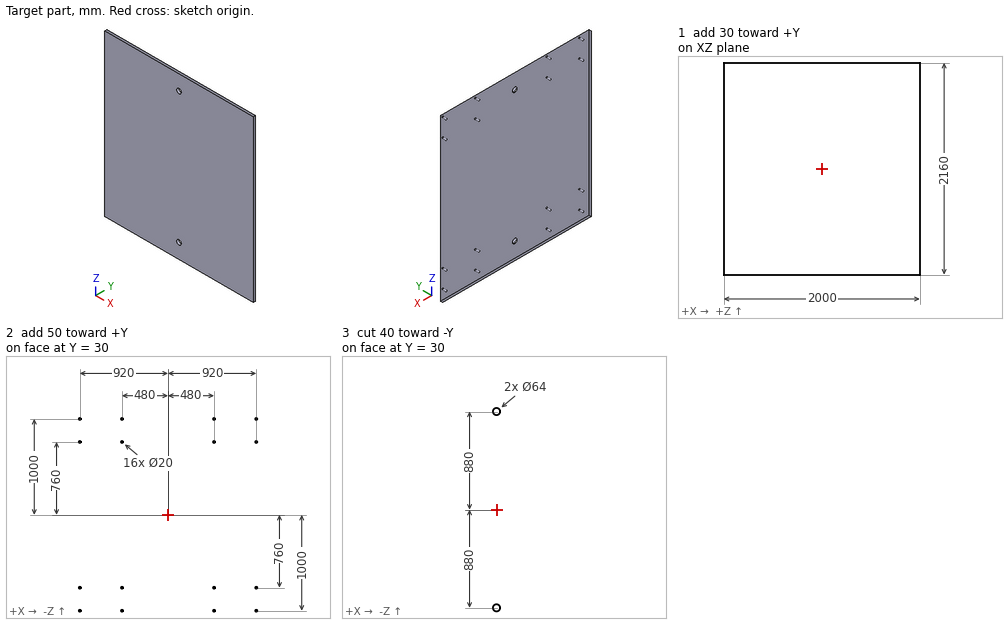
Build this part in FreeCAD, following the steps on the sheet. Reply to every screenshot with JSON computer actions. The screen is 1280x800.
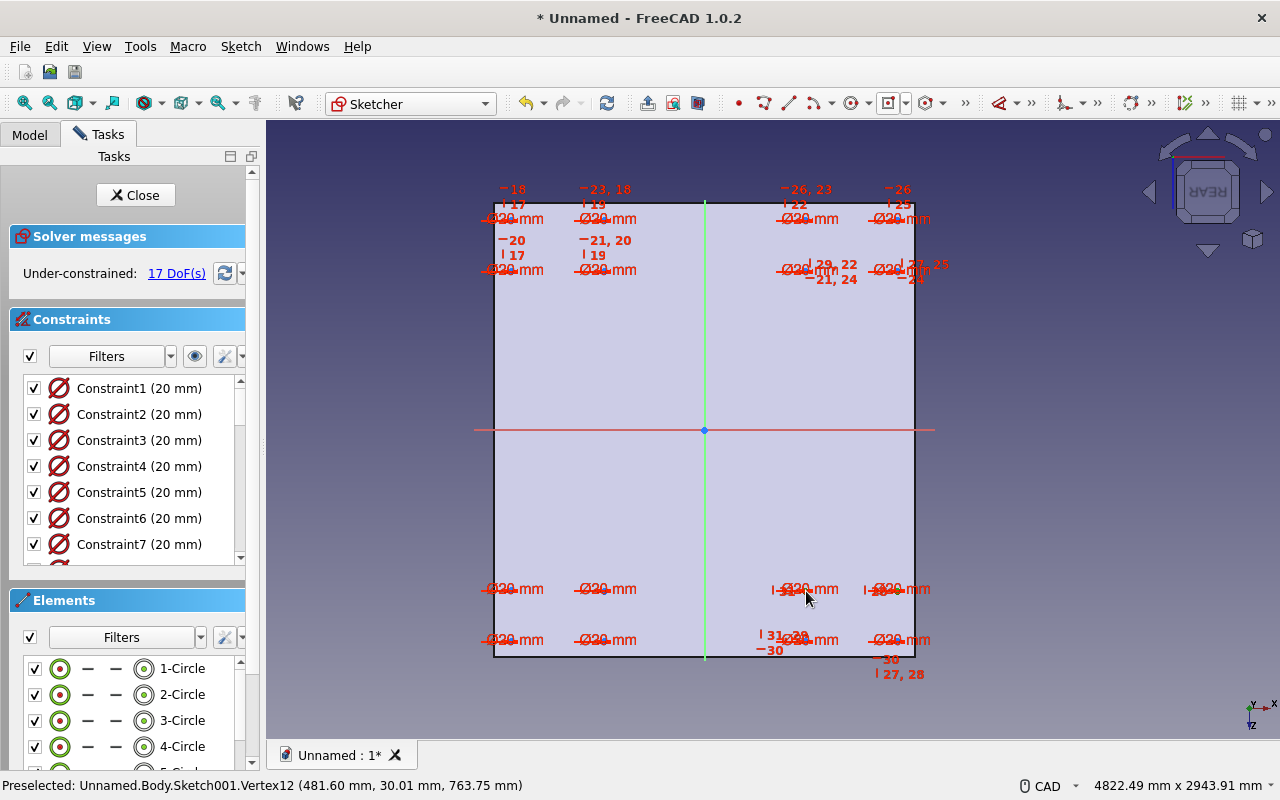
{"action": "key", "text": "h"}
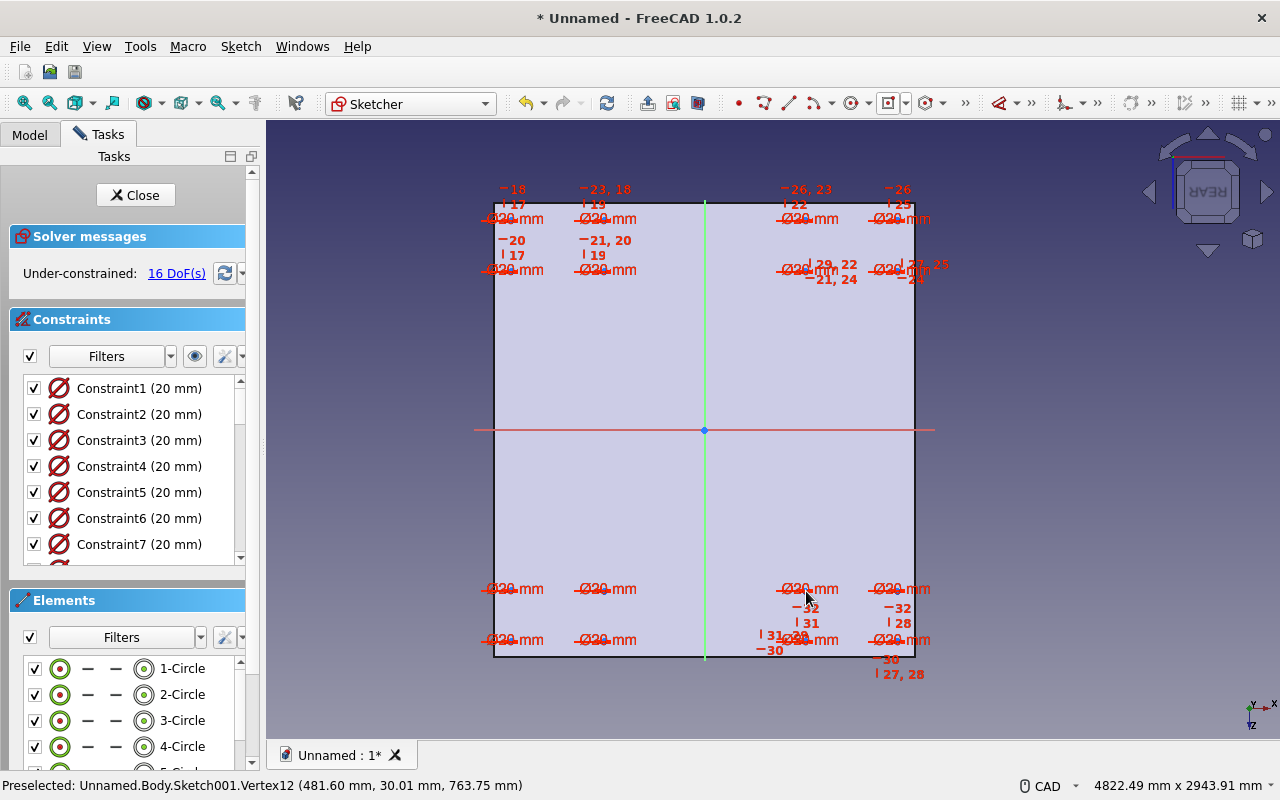
{"action": "left_click", "coordinate": [604, 272]}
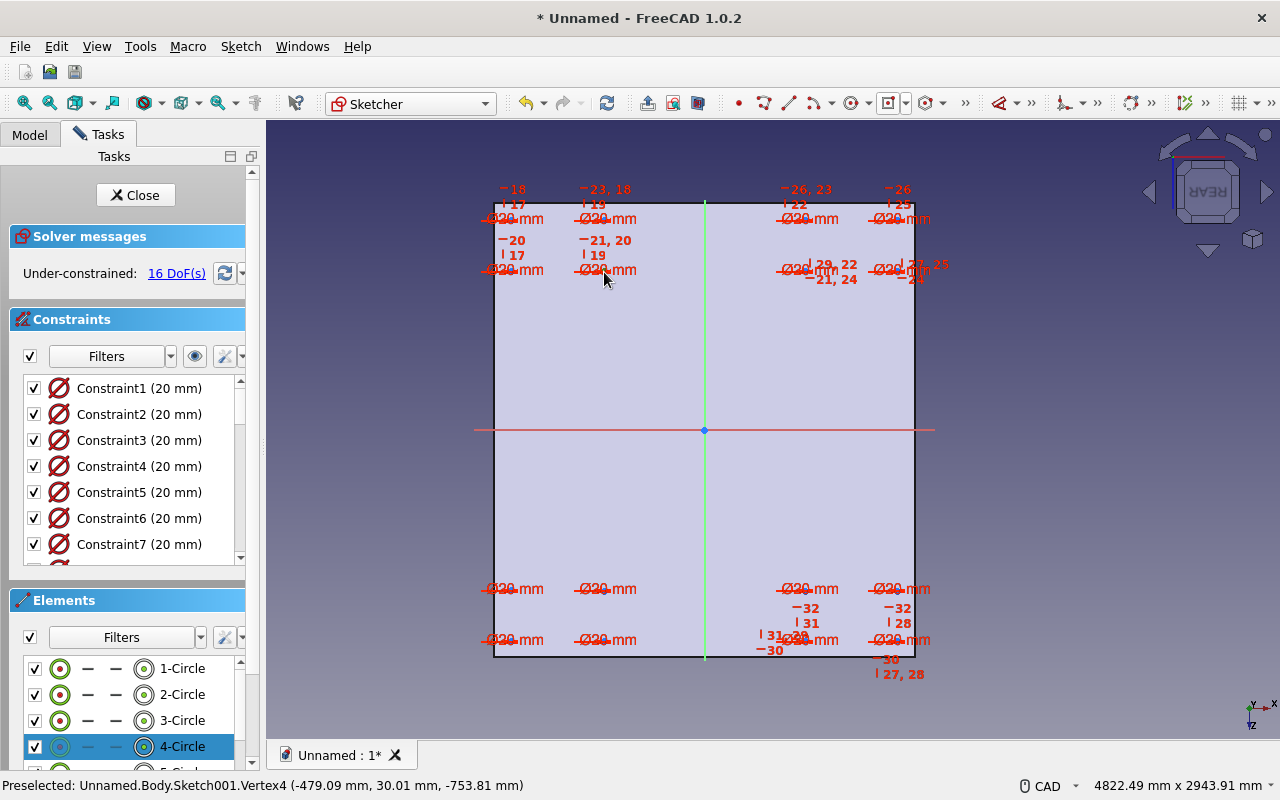
{"action": "left_click", "coordinate": [604, 591]}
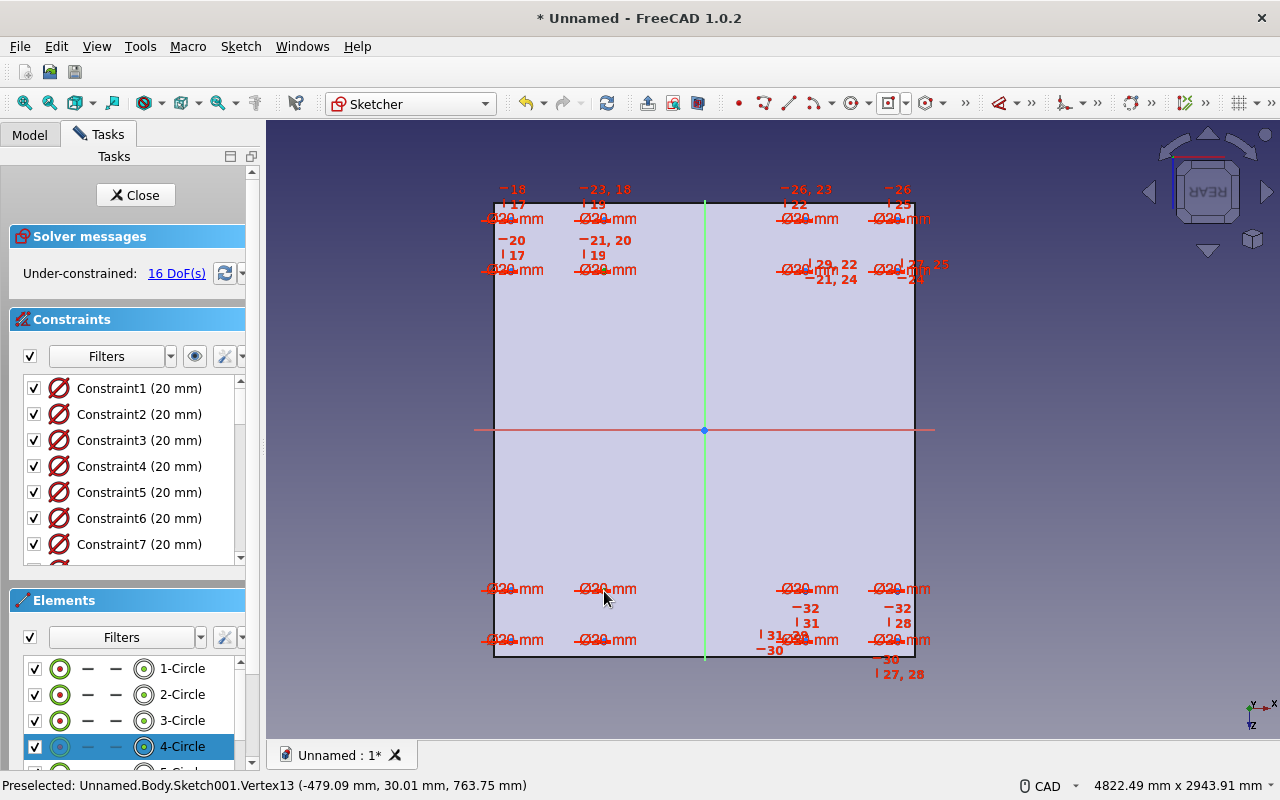
{"action": "key", "text": "v"}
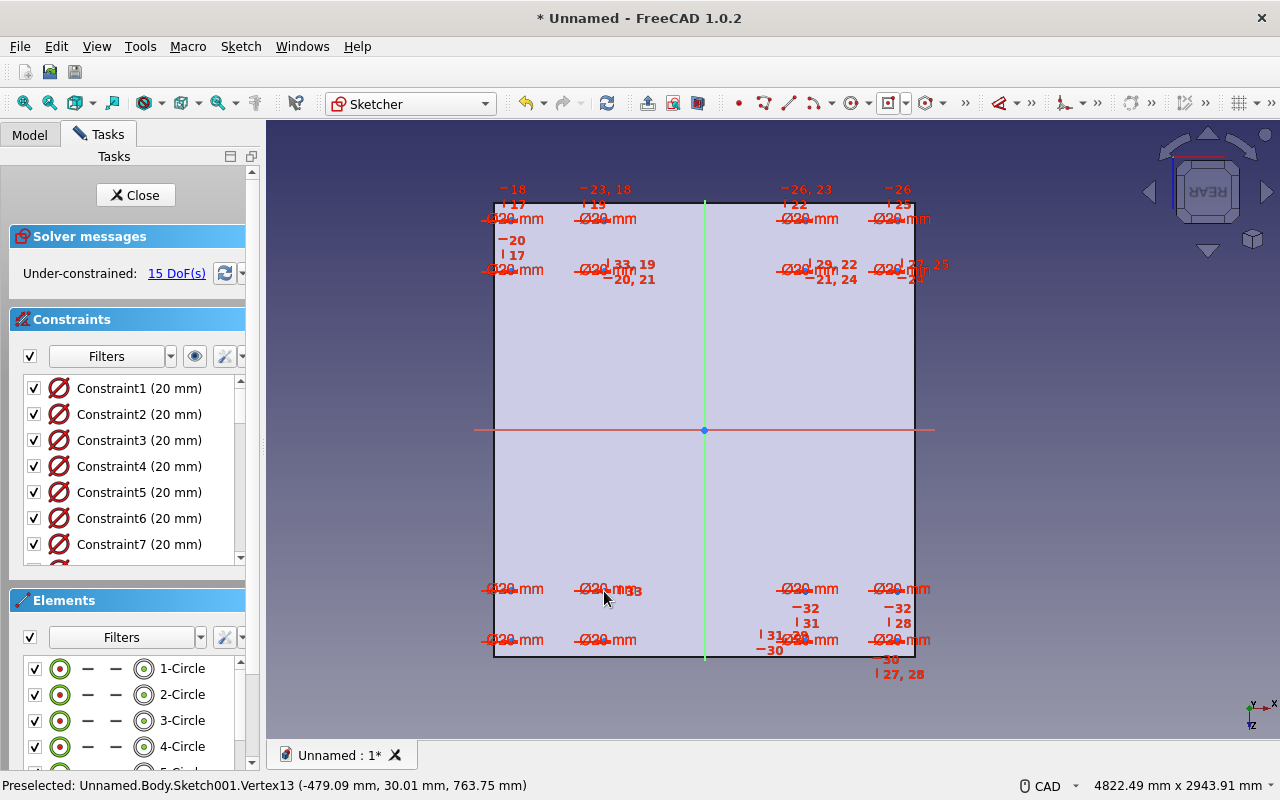
{"action": "left_click", "coordinate": [806, 591]}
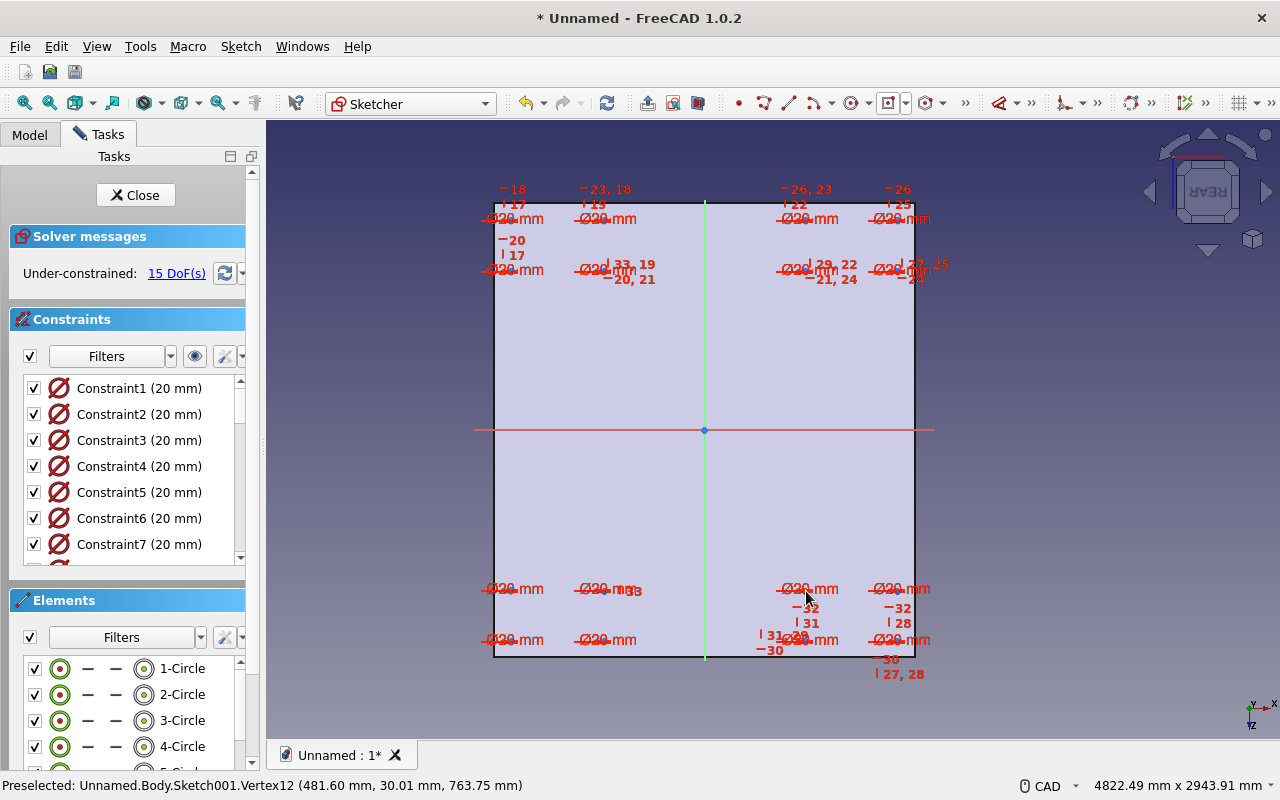
{"action": "left_click", "coordinate": [604, 591]}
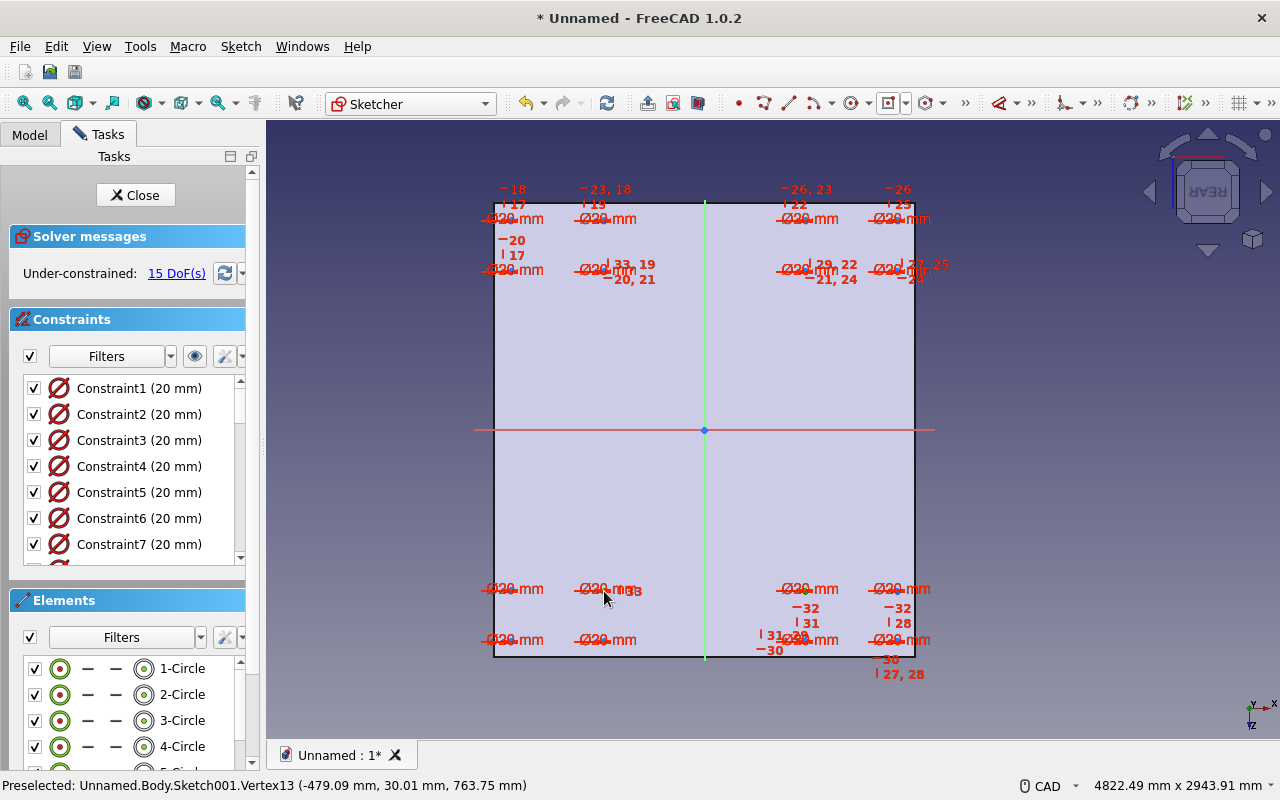
{"action": "key", "text": "h"}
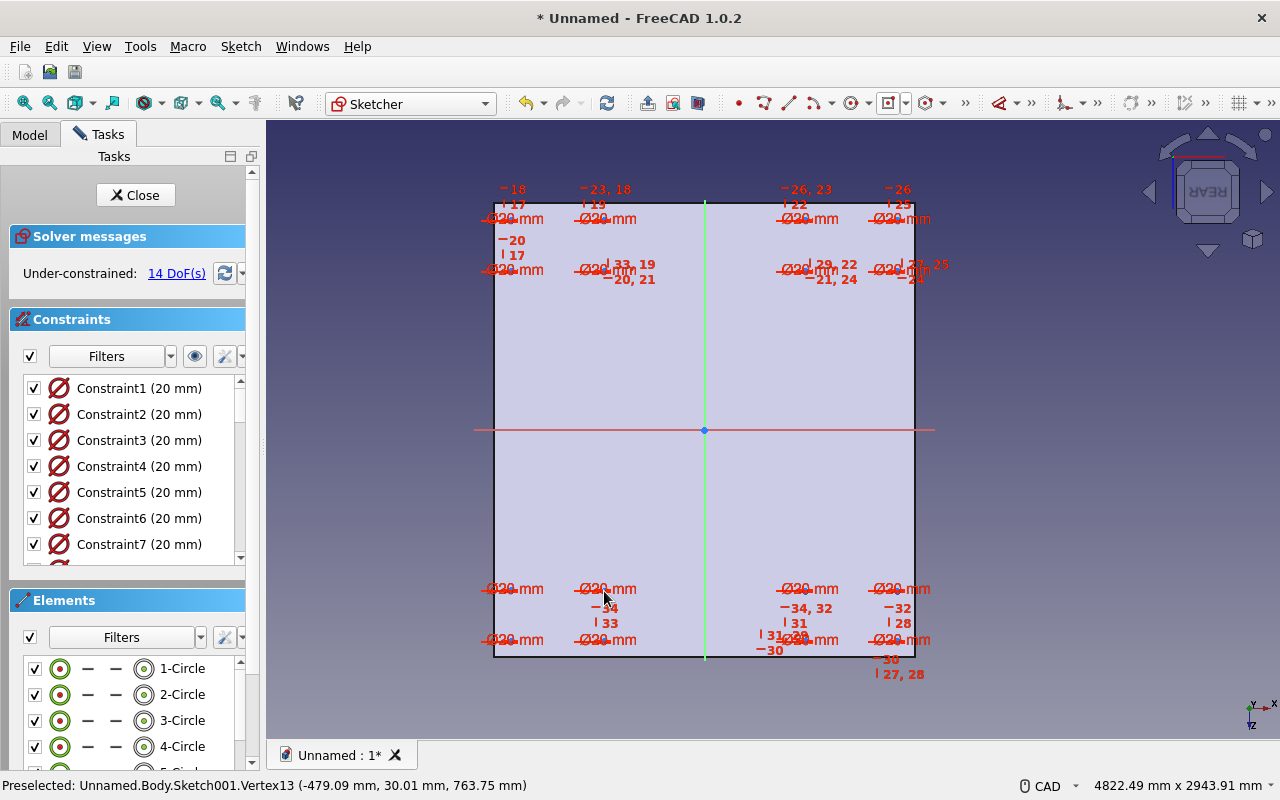
{"action": "left_click", "coordinate": [604, 591]}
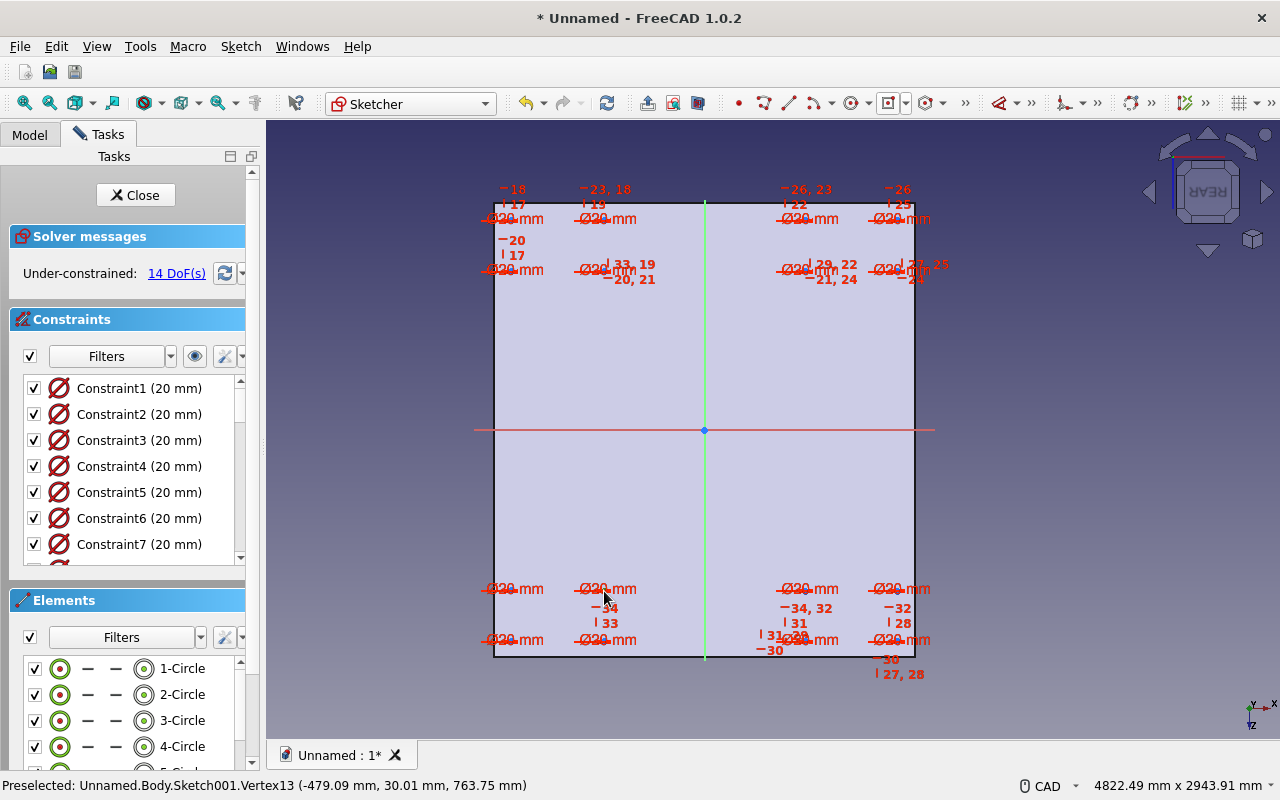
{"action": "left_click", "coordinate": [604, 642]}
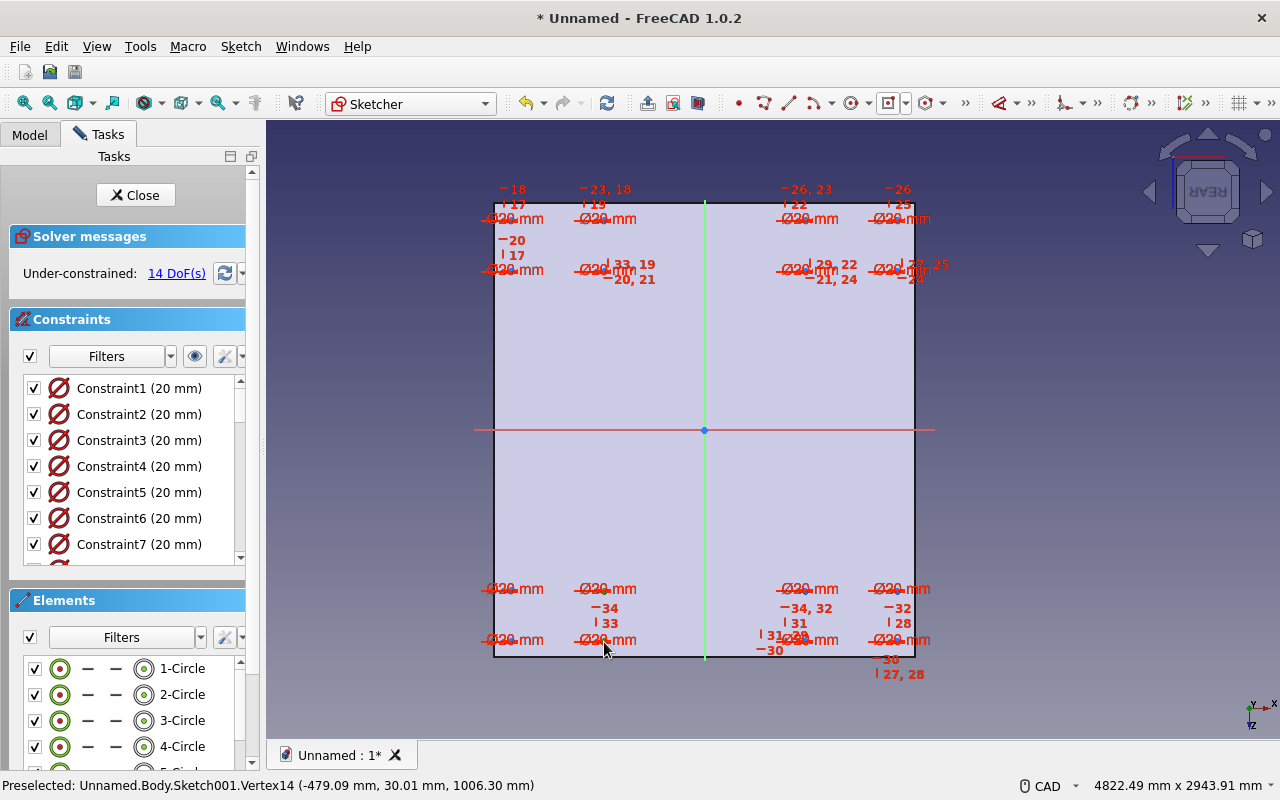
{"action": "key", "text": "v"}